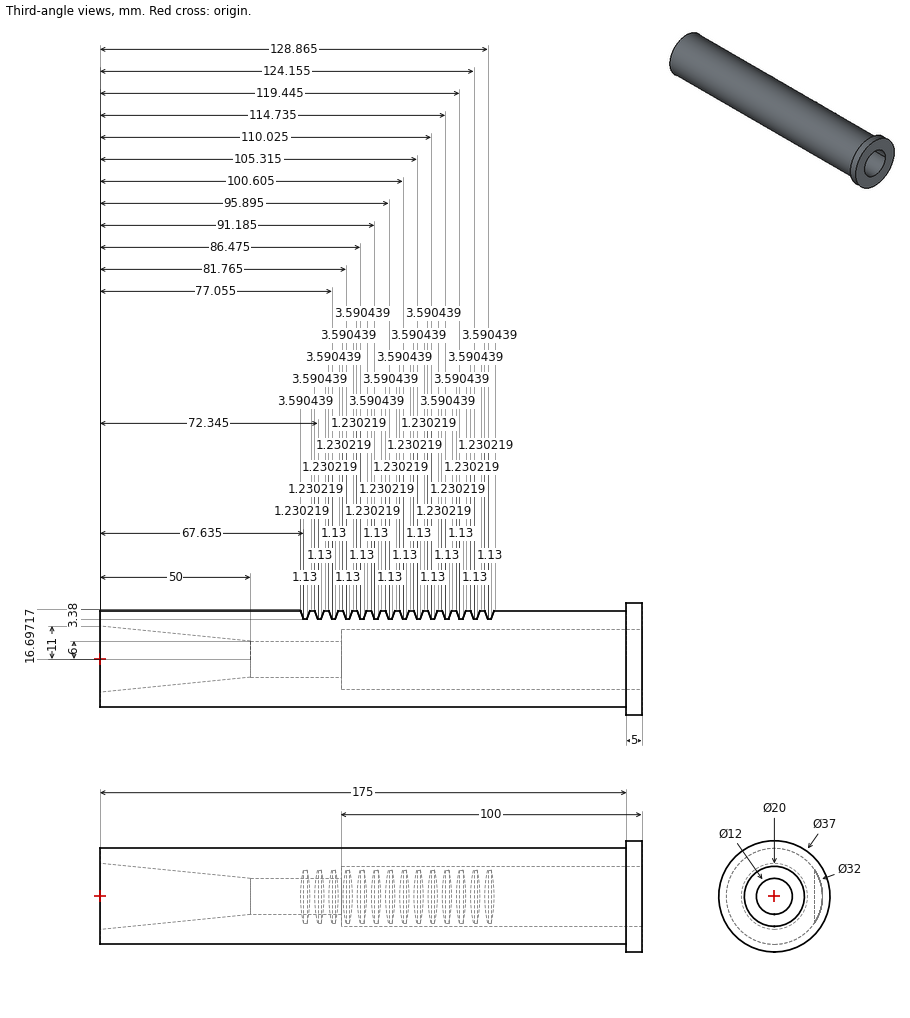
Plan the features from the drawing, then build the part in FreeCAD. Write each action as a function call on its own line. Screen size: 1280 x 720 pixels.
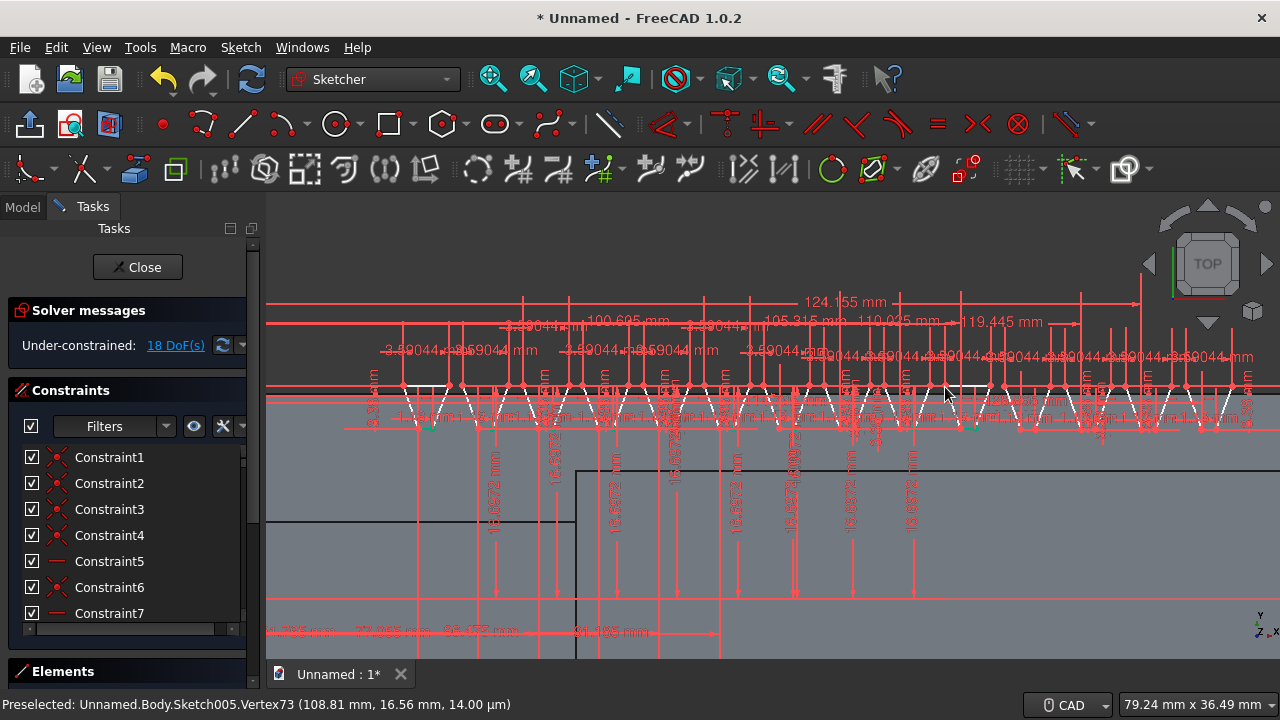
click(1005, 386)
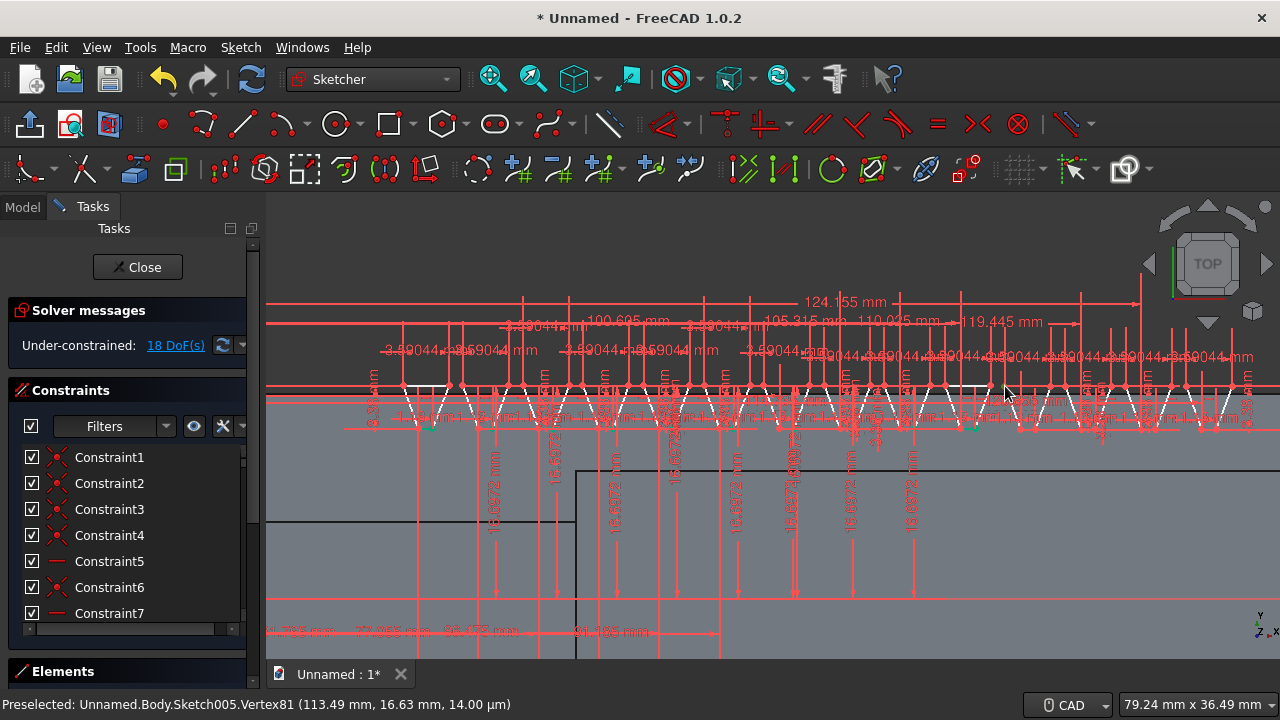
key(i)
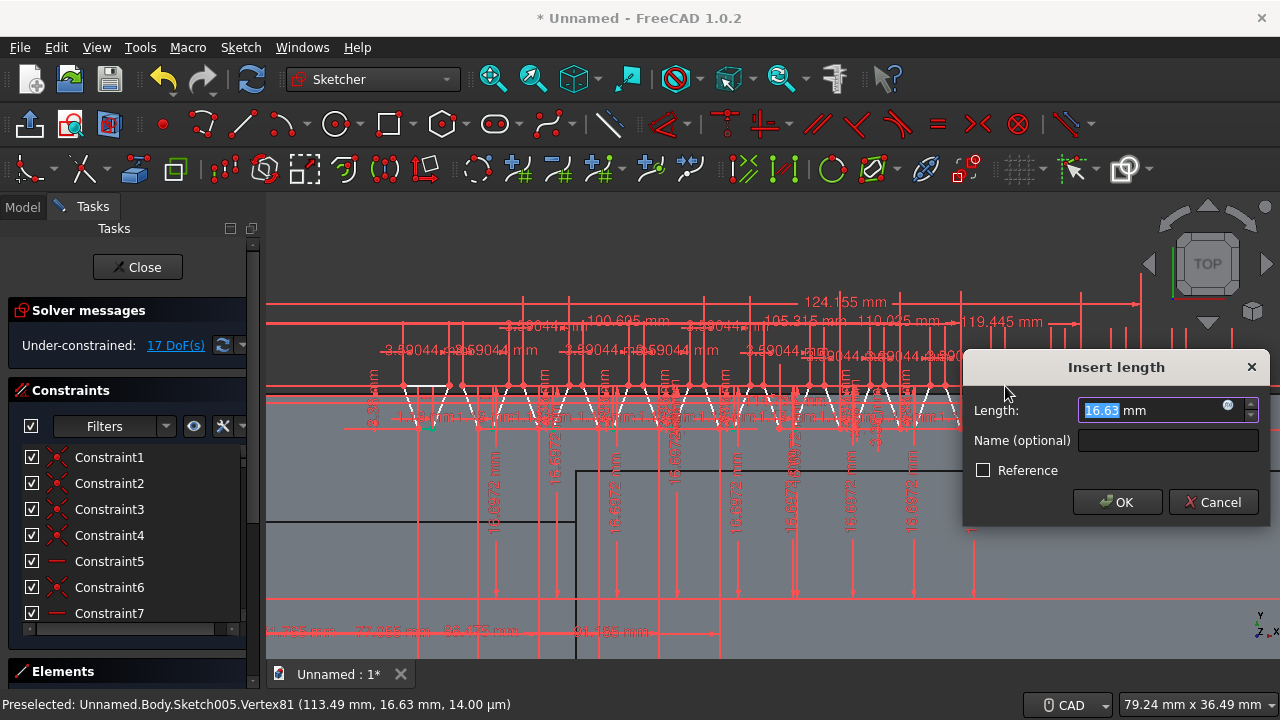
text(16.69717)
key(Return)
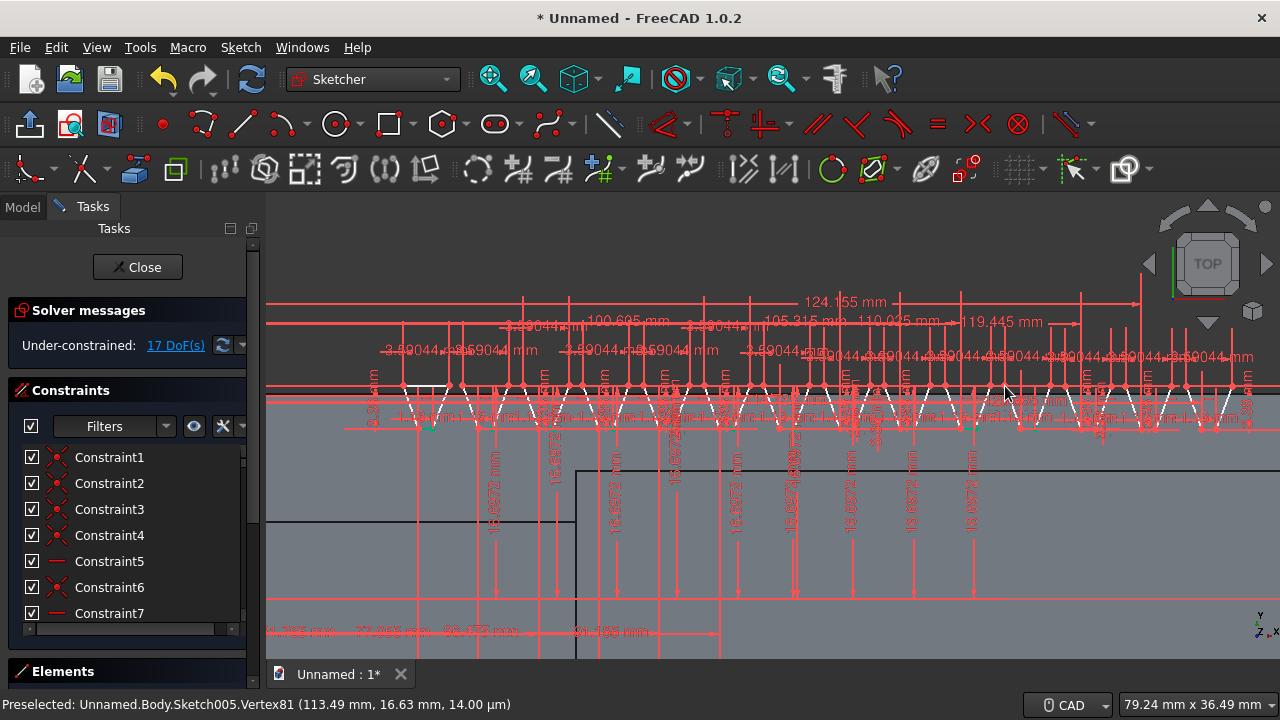
click(1065, 386)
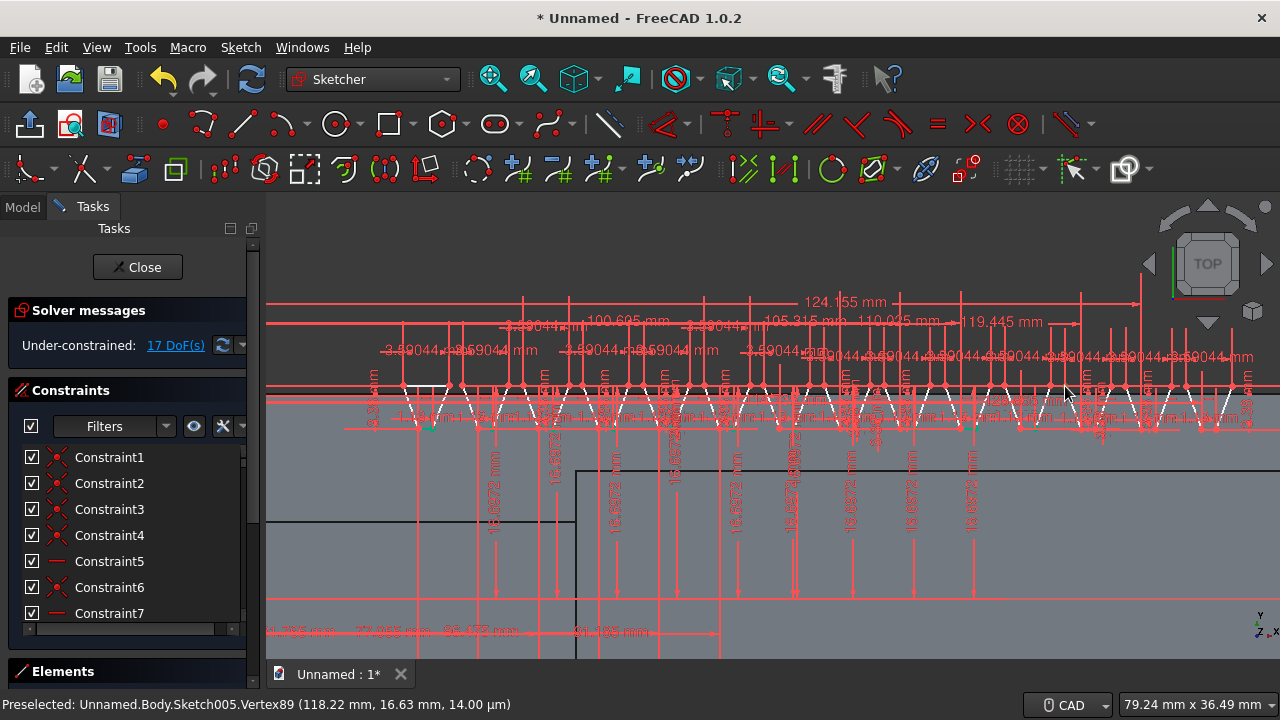
key(i)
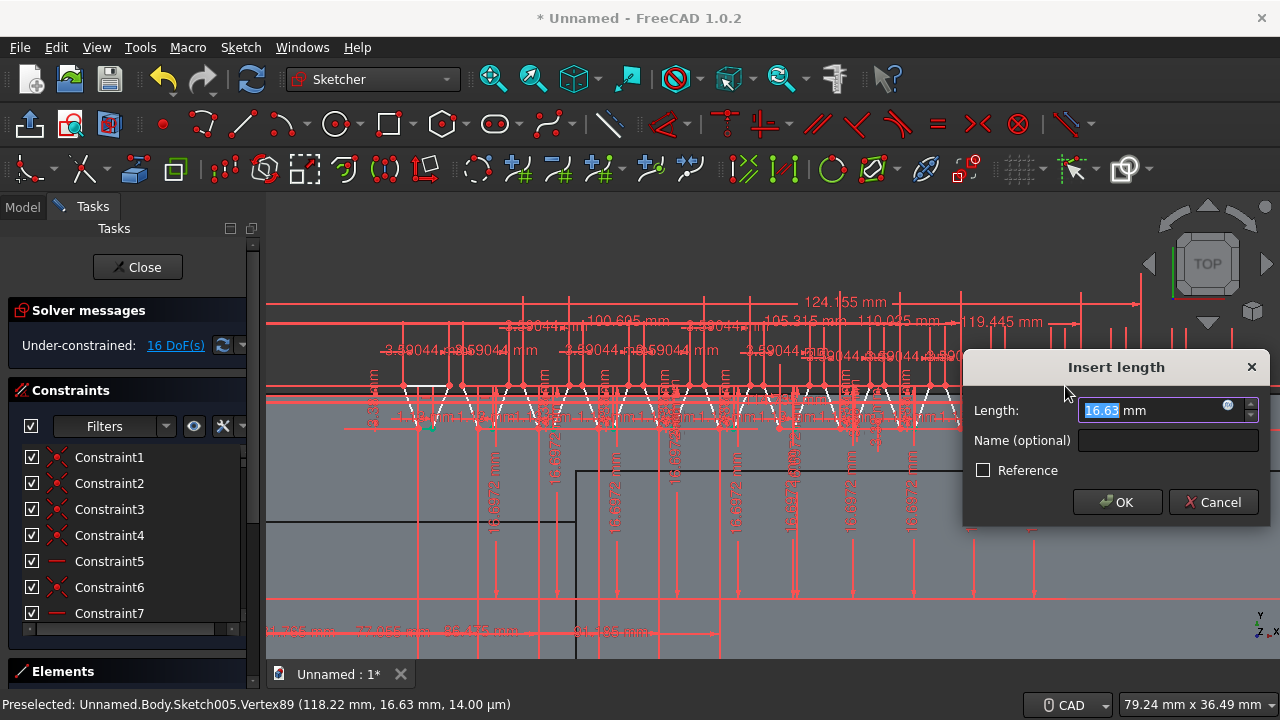
text(16.69717)
key(Return)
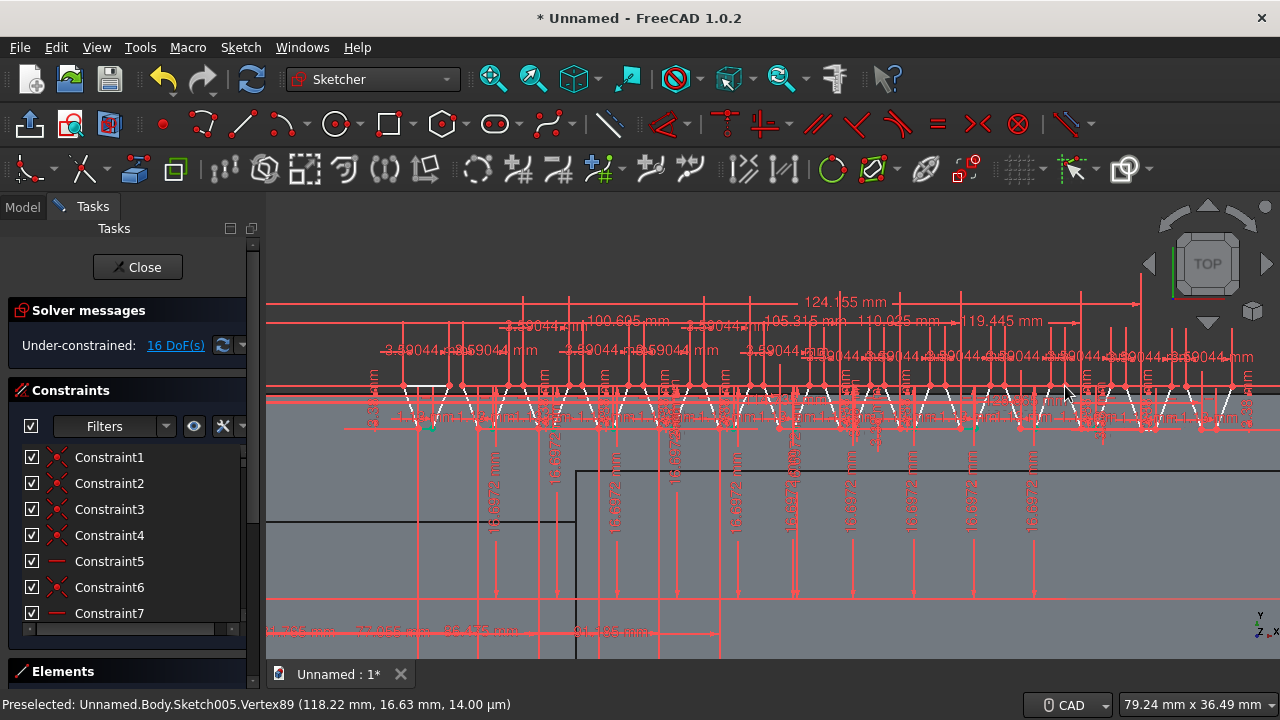
scroll(886, 387, down, 5)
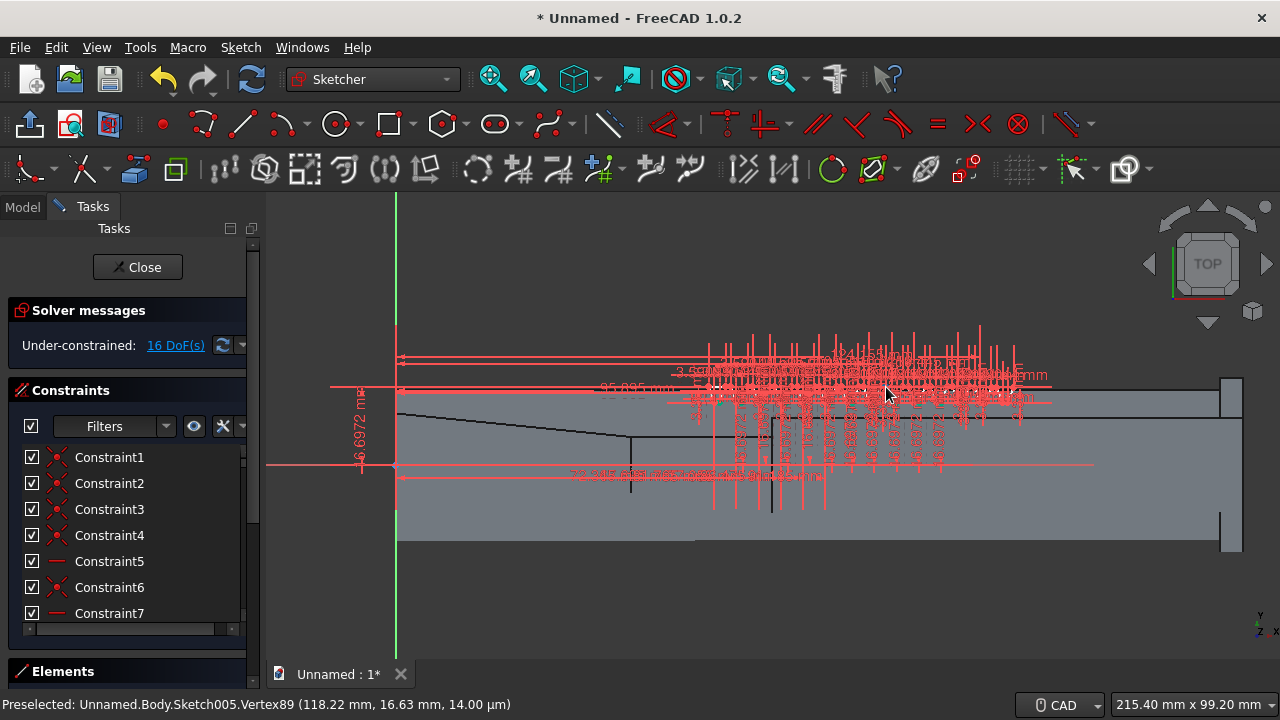
scroll(975, 387, up, 5)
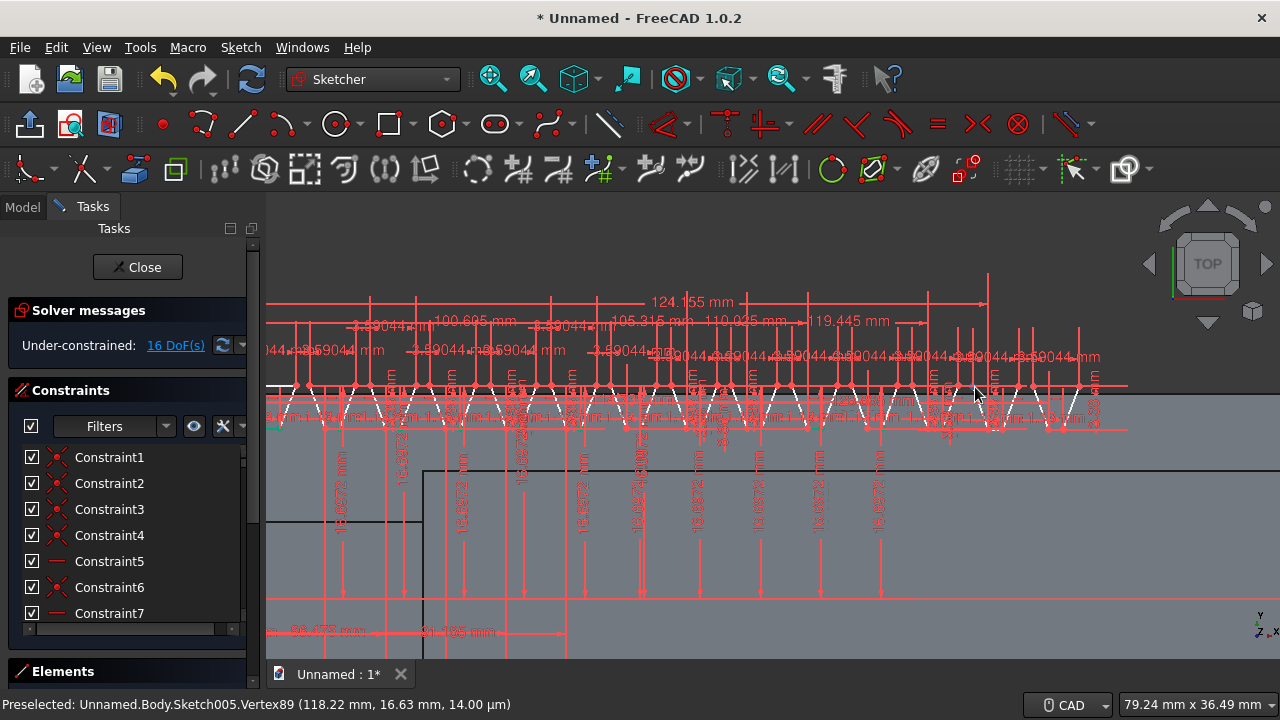
click(973, 386)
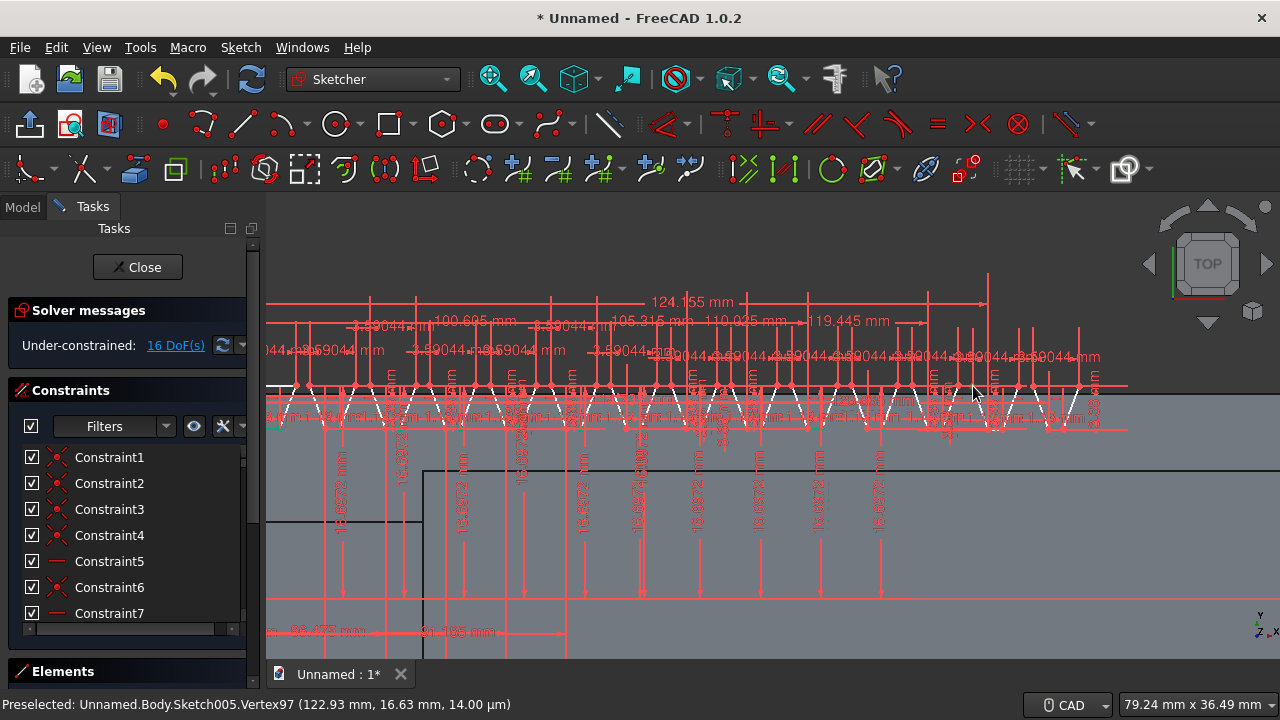
key(i)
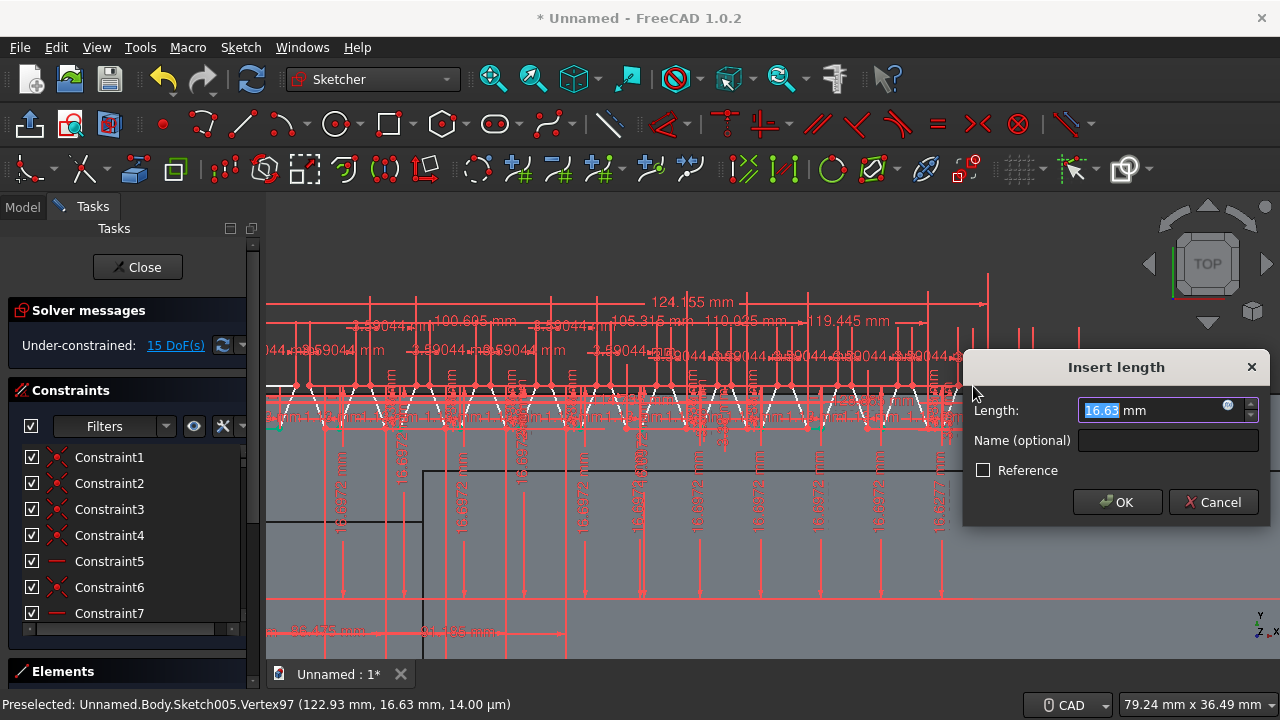
text(16.69717)
key(Return)